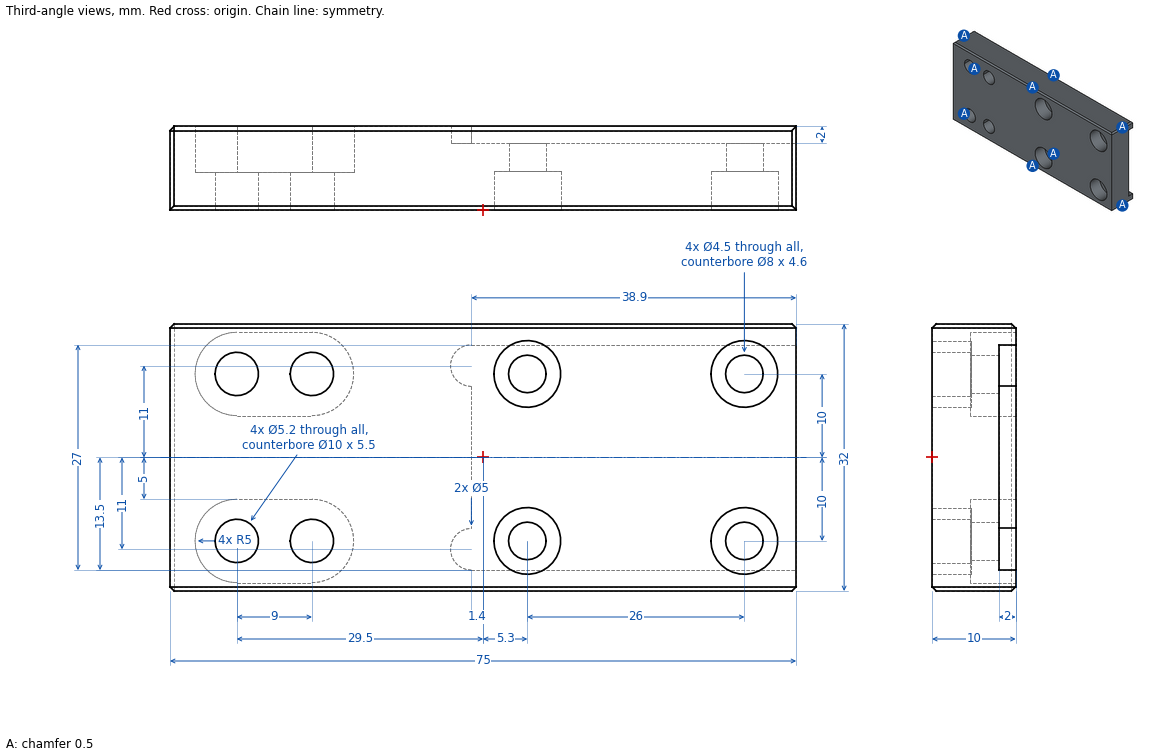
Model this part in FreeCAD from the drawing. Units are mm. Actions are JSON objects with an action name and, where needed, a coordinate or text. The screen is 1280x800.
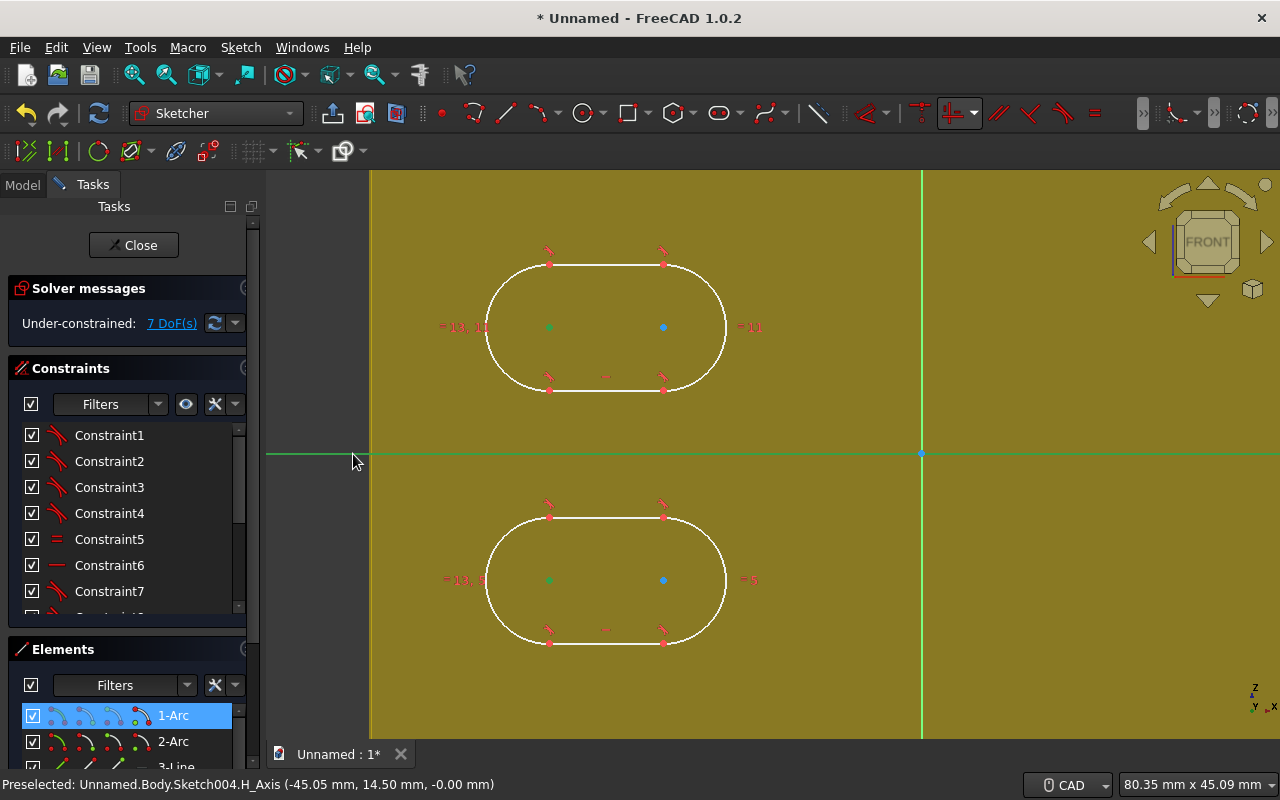
{"action": "key", "text": "s"}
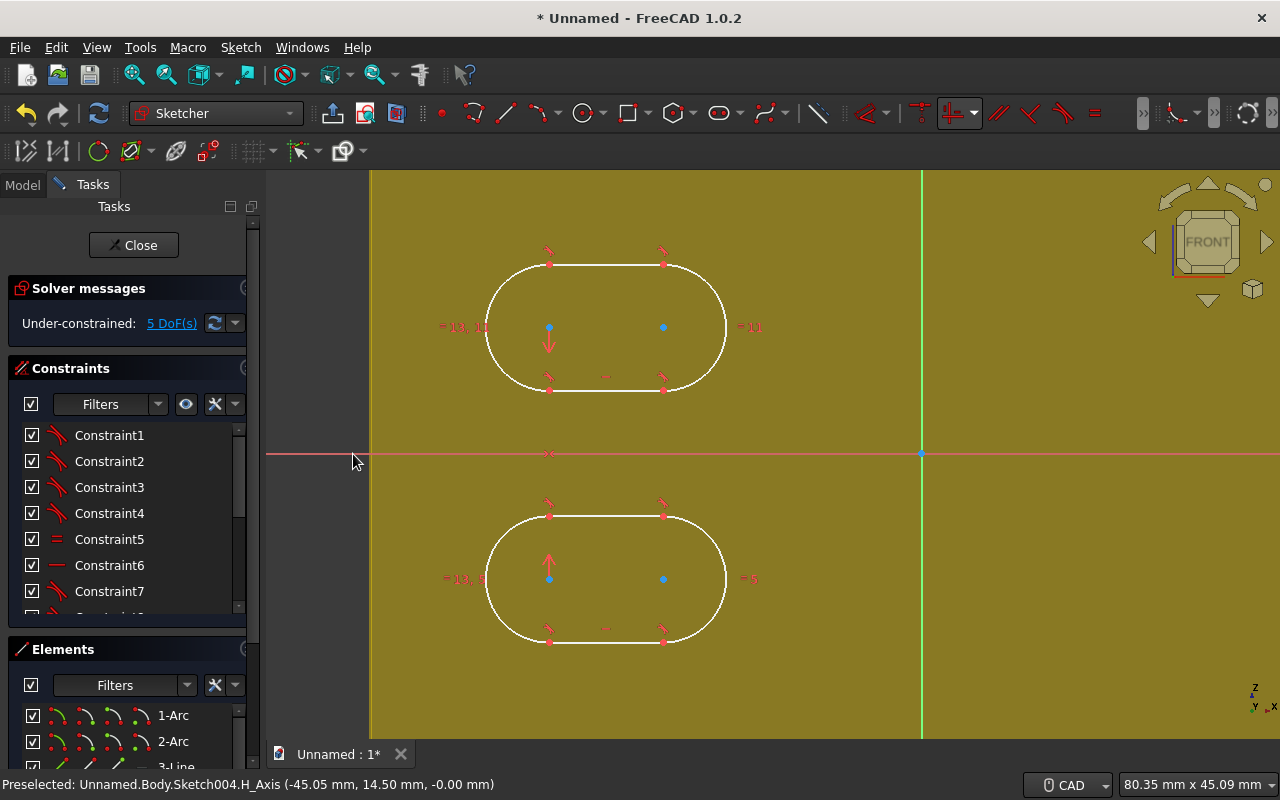
{"action": "left_click", "coordinate": [866, 114]}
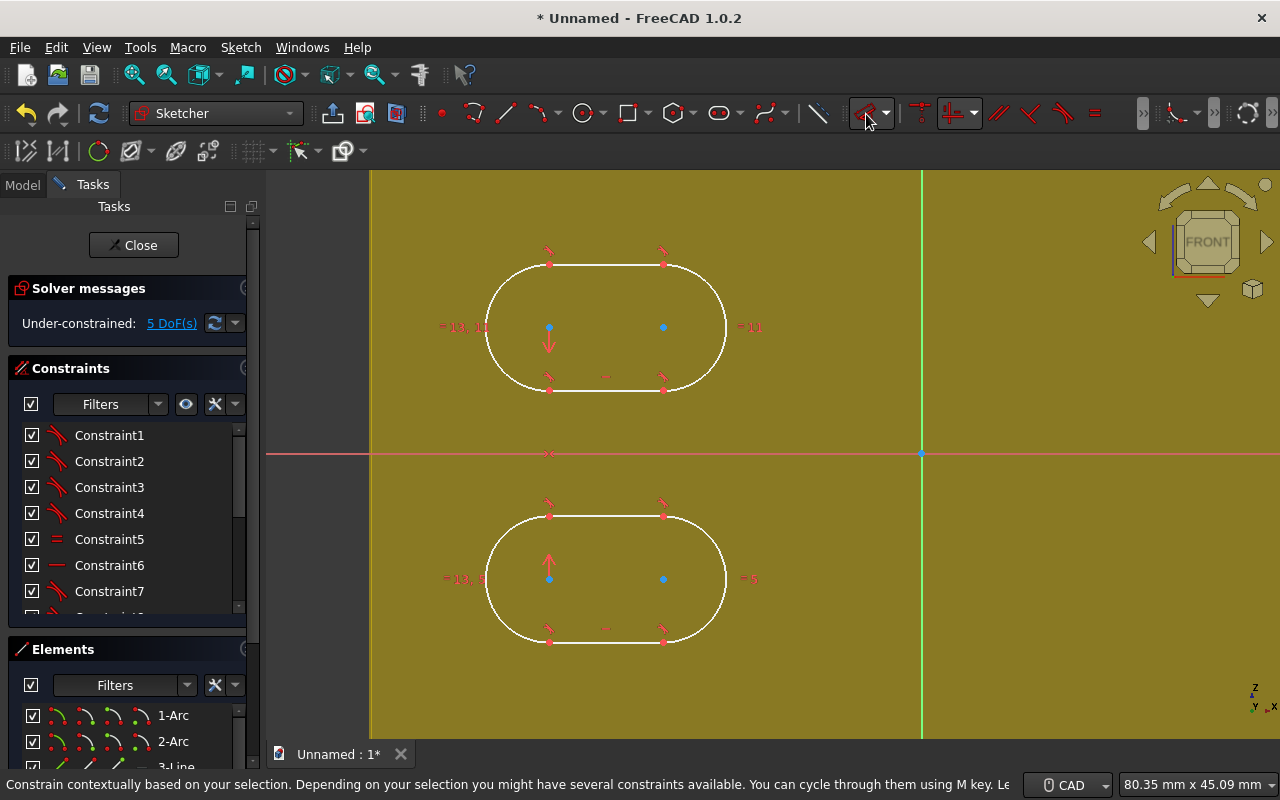
{"action": "left_click", "coordinate": [498, 542]}
{"action": "left_click", "coordinate": [472, 523]}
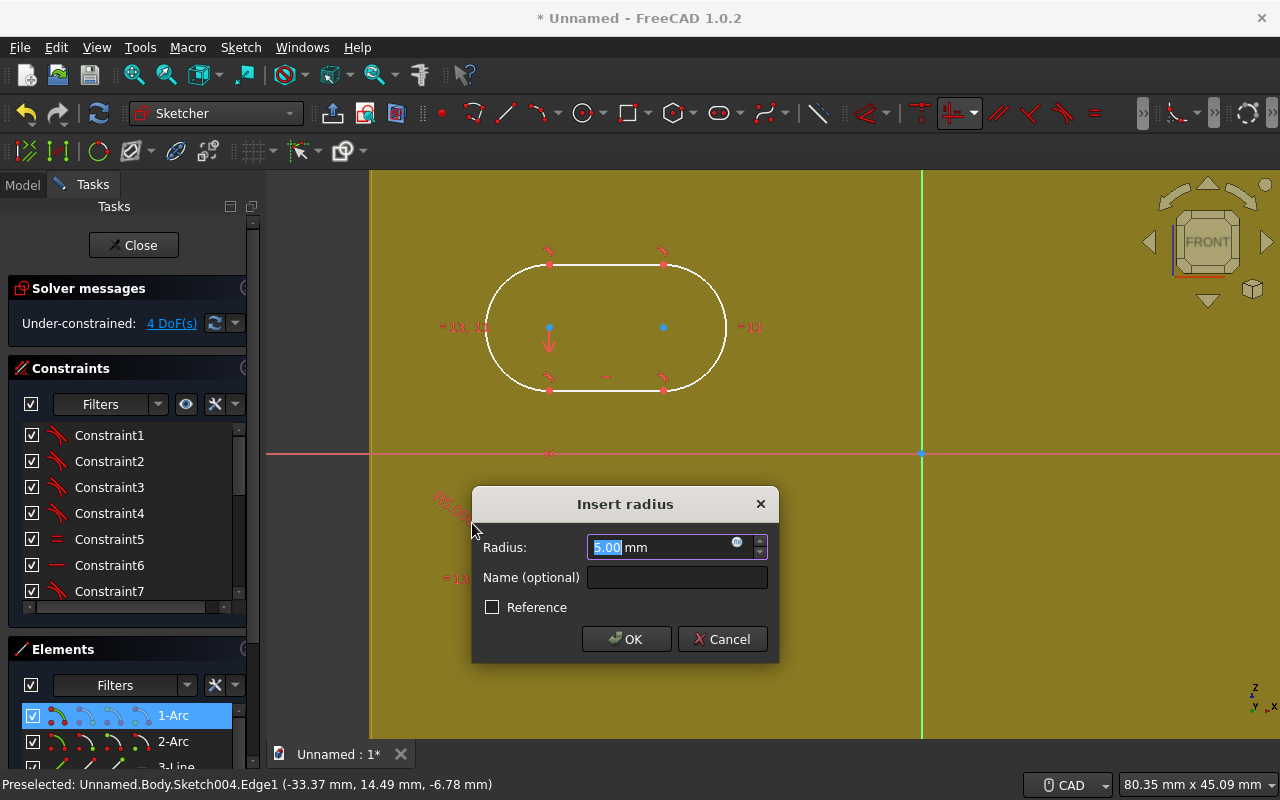
{"action": "type", "text": "5"}
{"action": "key", "text": "Return"}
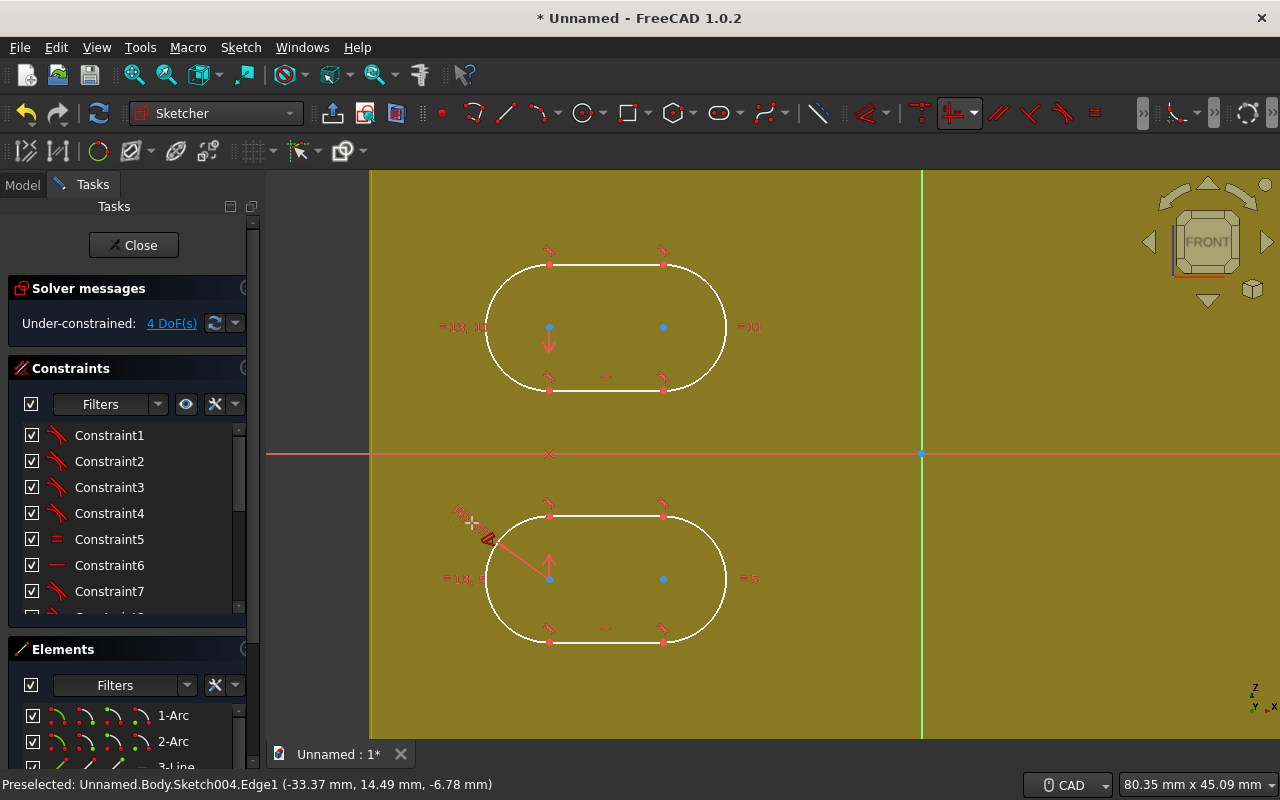
{"action": "left_click", "coordinate": [583, 516]}
{"action": "left_click", "coordinate": [606, 550]}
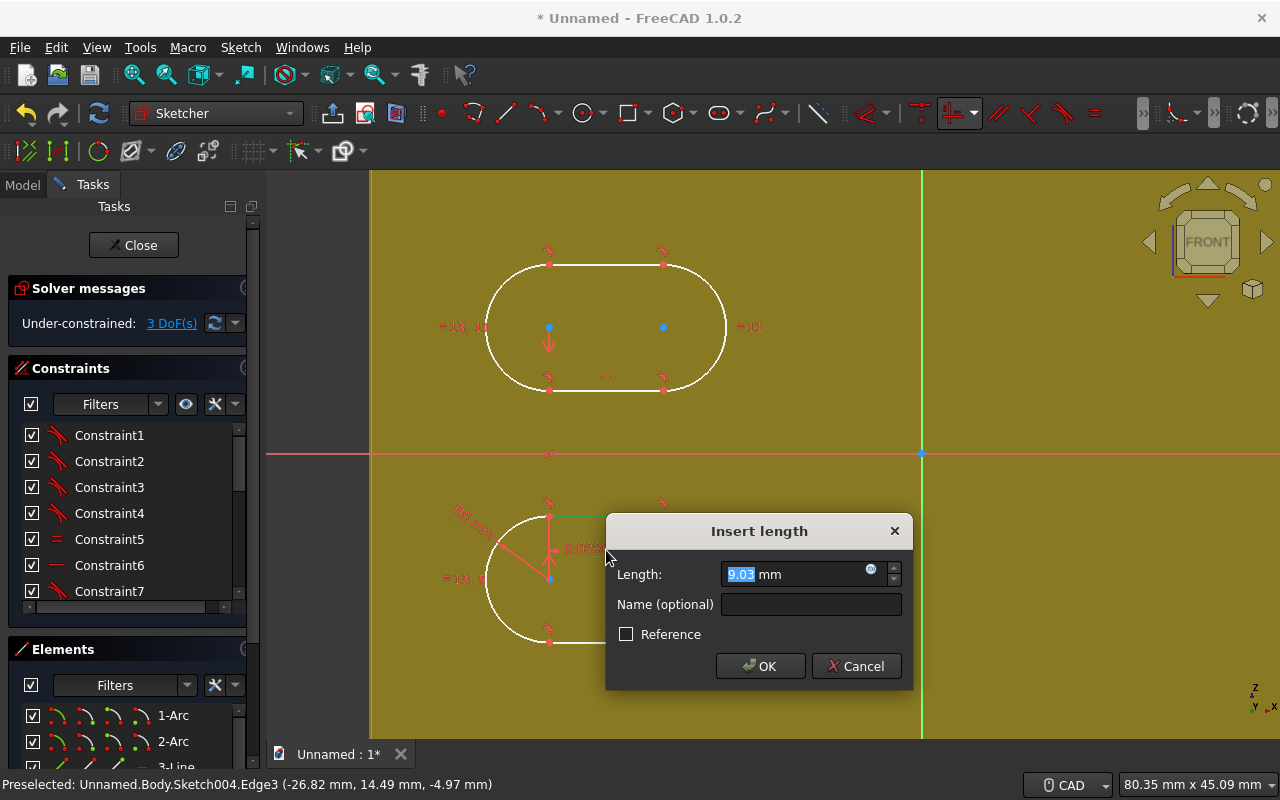
{"action": "type", "text": "9"}
{"action": "key", "text": "Return"}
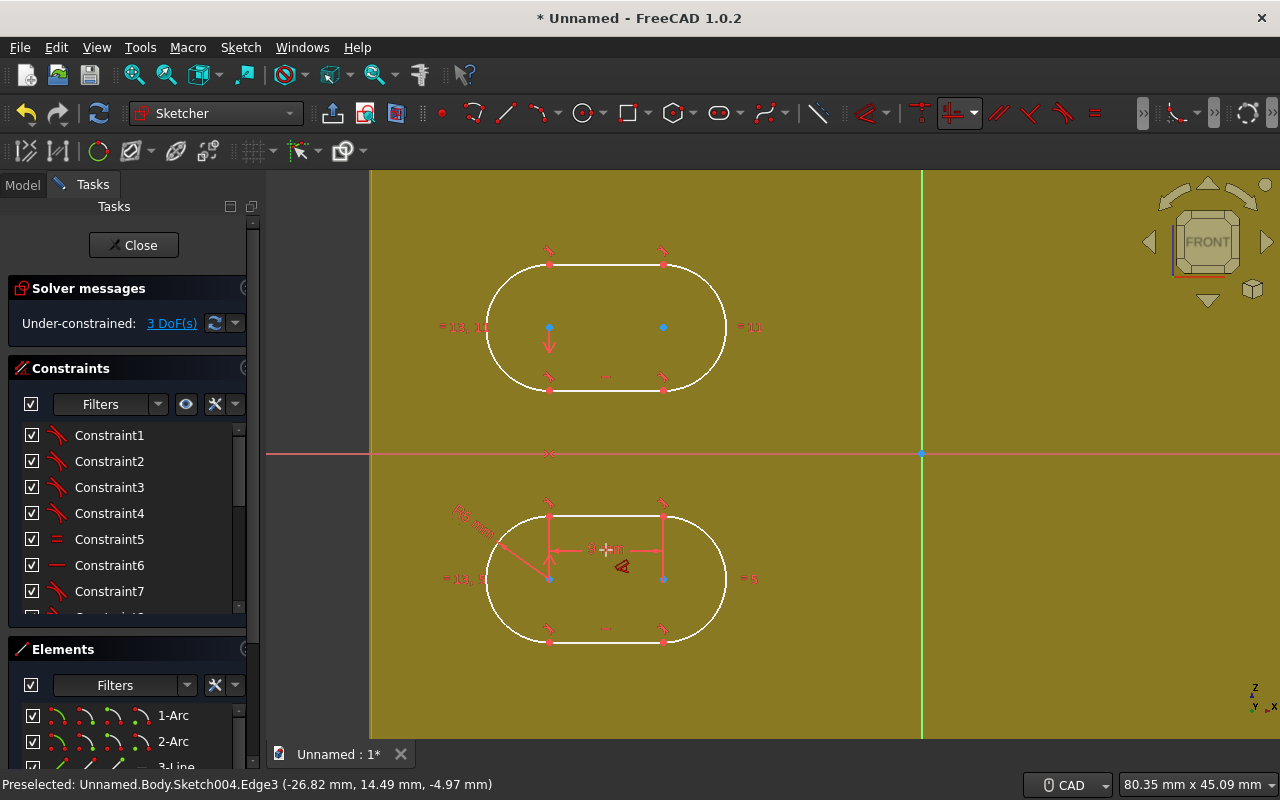
{"action": "left_click", "coordinate": [583, 265]}
{"action": "left_click", "coordinate": [606, 231]}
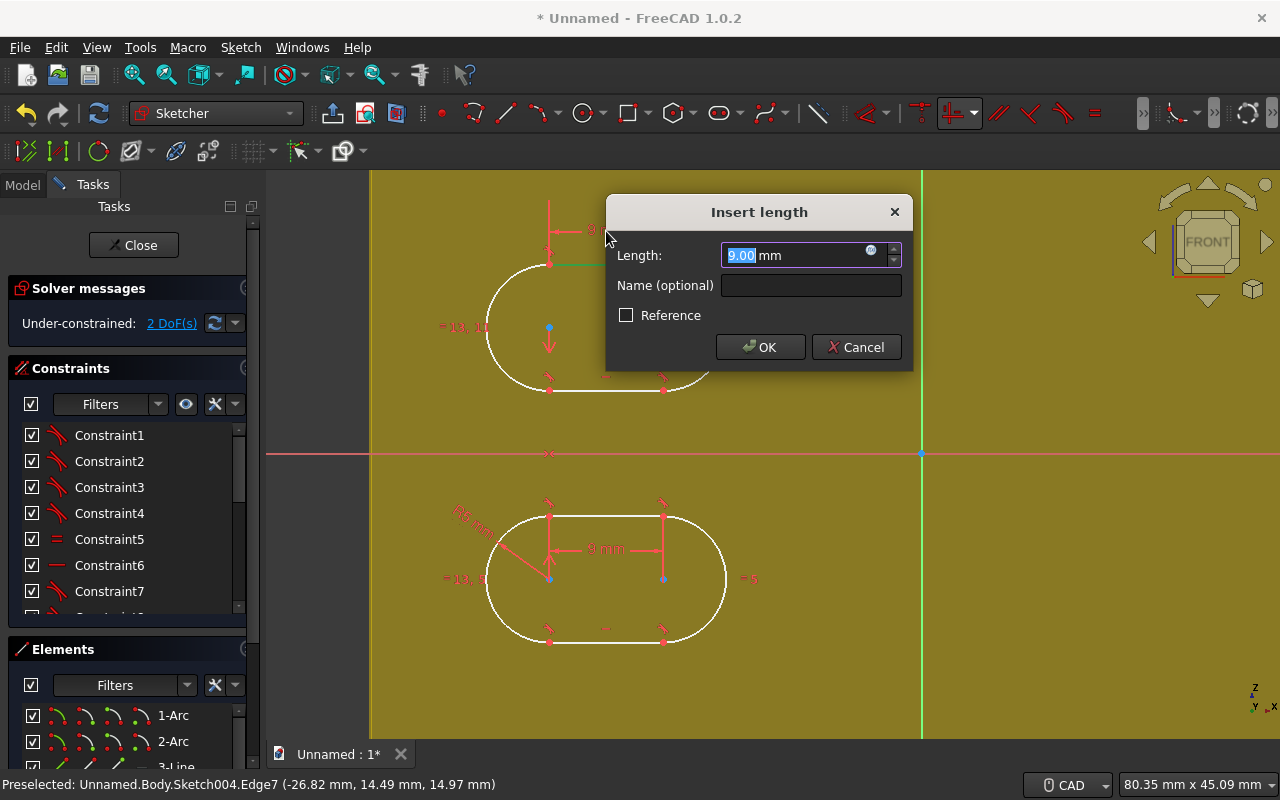
{"action": "type", "text": "9"}
{"action": "key", "text": "Return"}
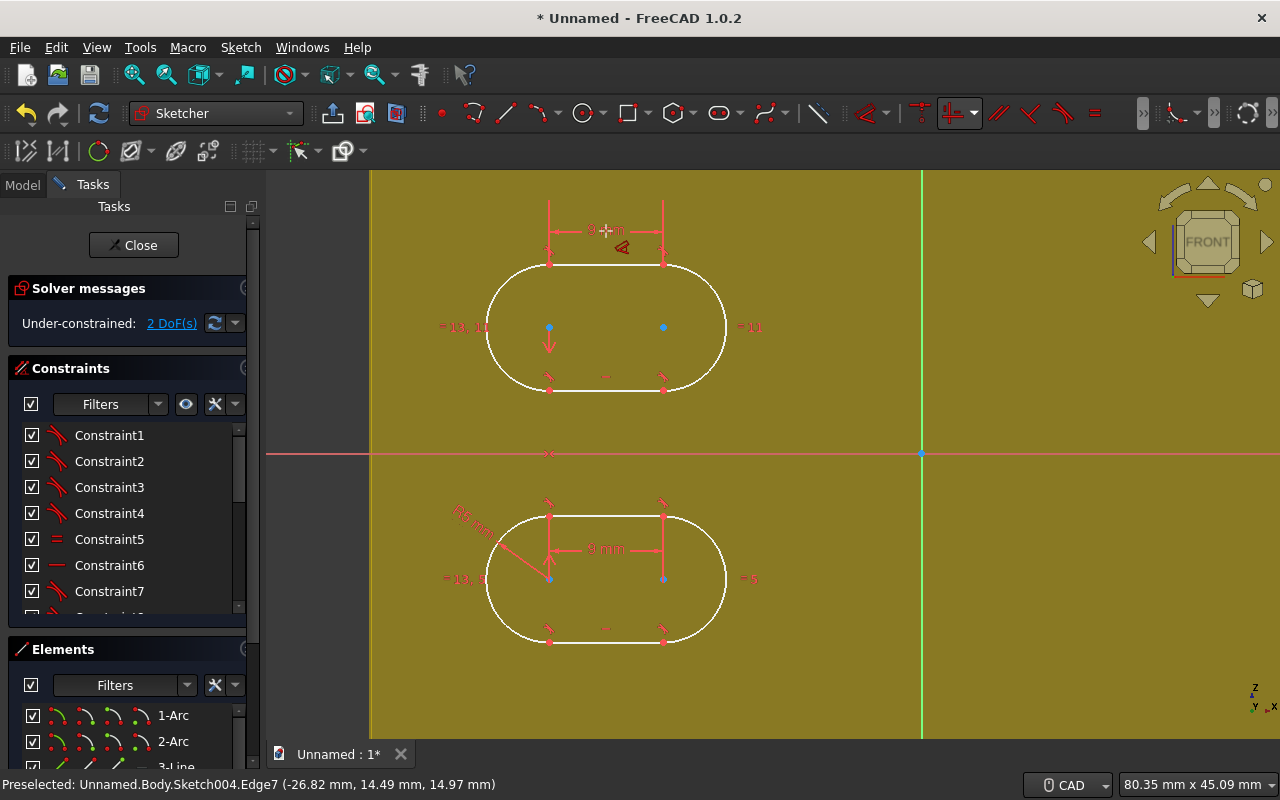
{"action": "left_click", "coordinate": [549, 516]}
{"action": "left_click", "coordinate": [956, 485]}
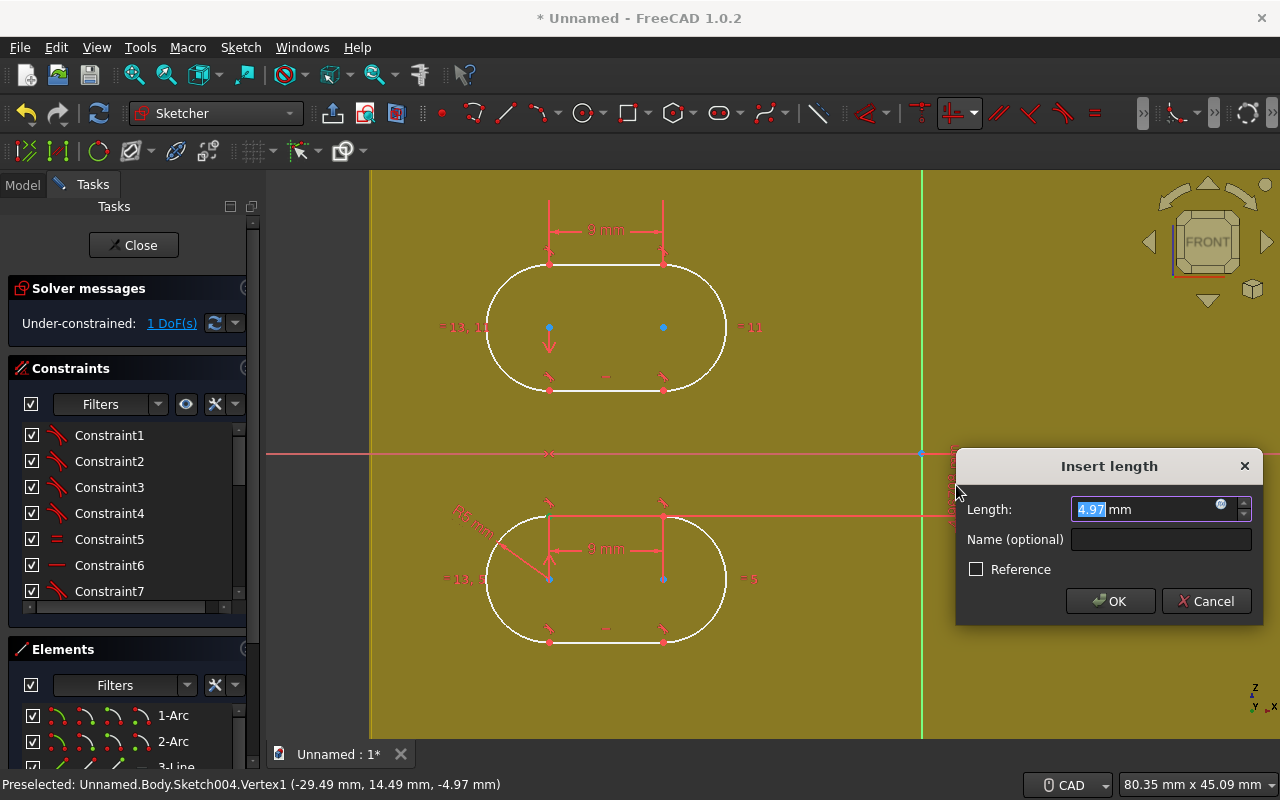
{"action": "type", "text": "5"}
{"action": "key", "text": "Return"}